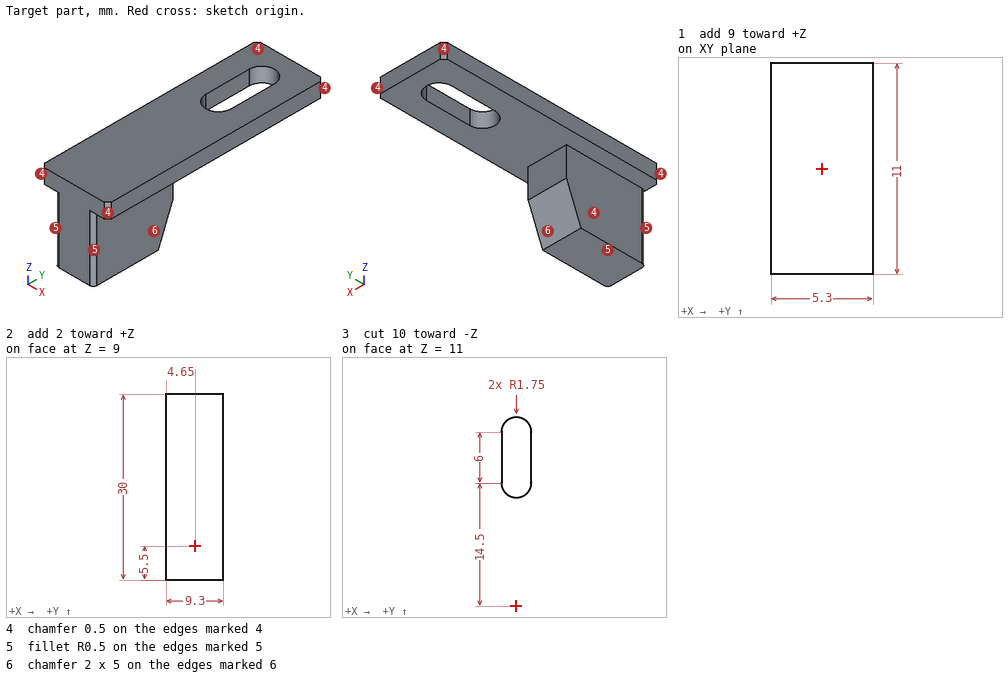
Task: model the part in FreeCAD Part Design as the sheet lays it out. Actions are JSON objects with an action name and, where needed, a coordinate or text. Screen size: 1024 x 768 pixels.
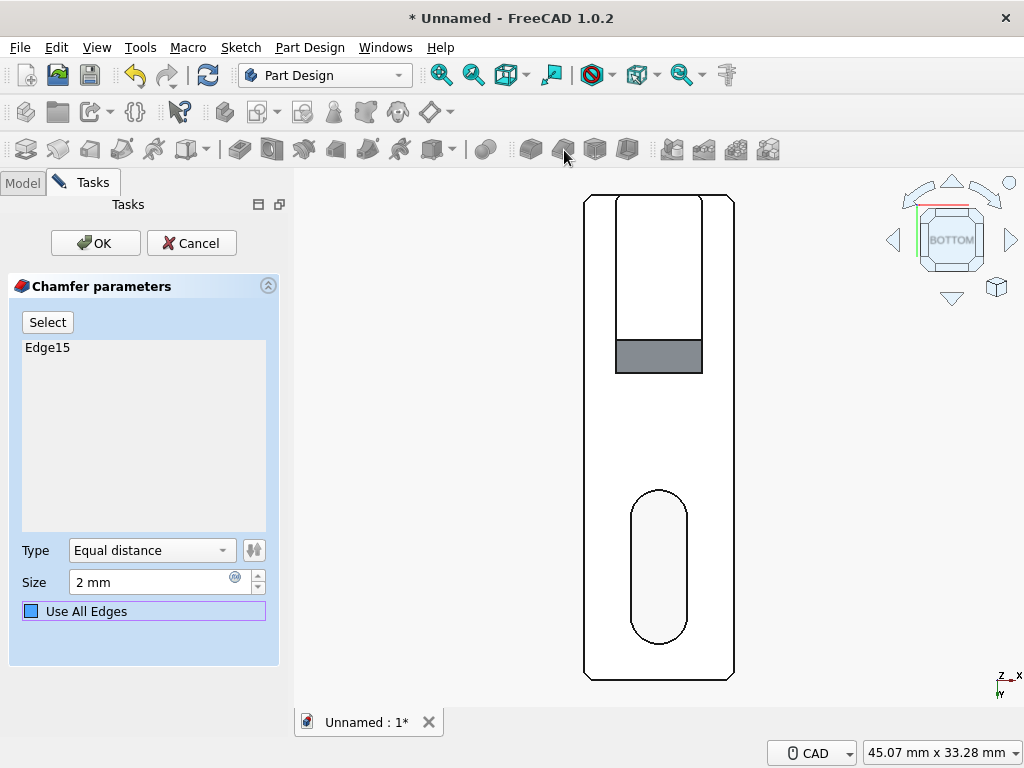
{"action": "left_click", "coordinate": [153, 550]}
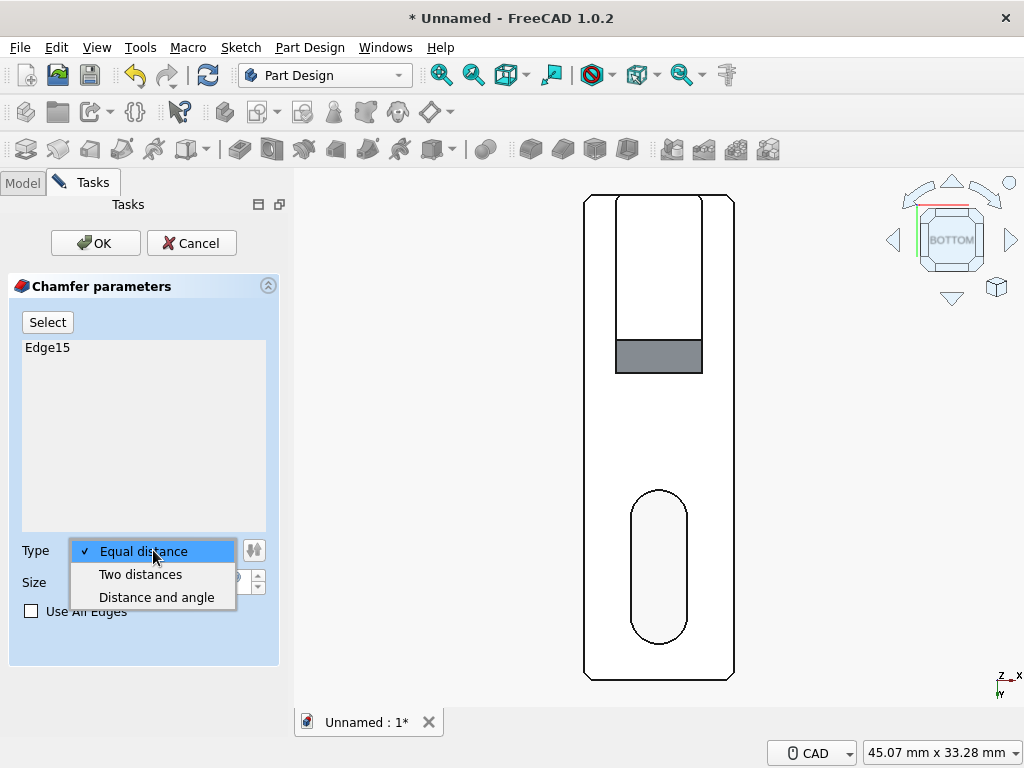
{"action": "left_click", "coordinate": [152, 574]}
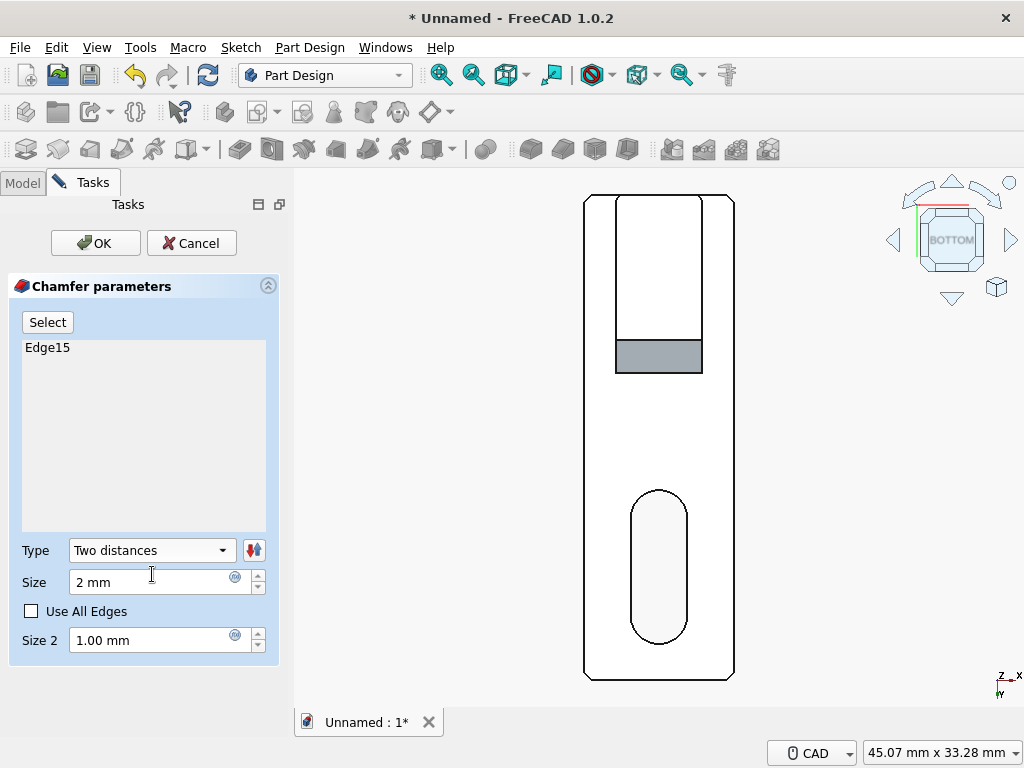
{"action": "triple_click", "coordinate": [160, 640]}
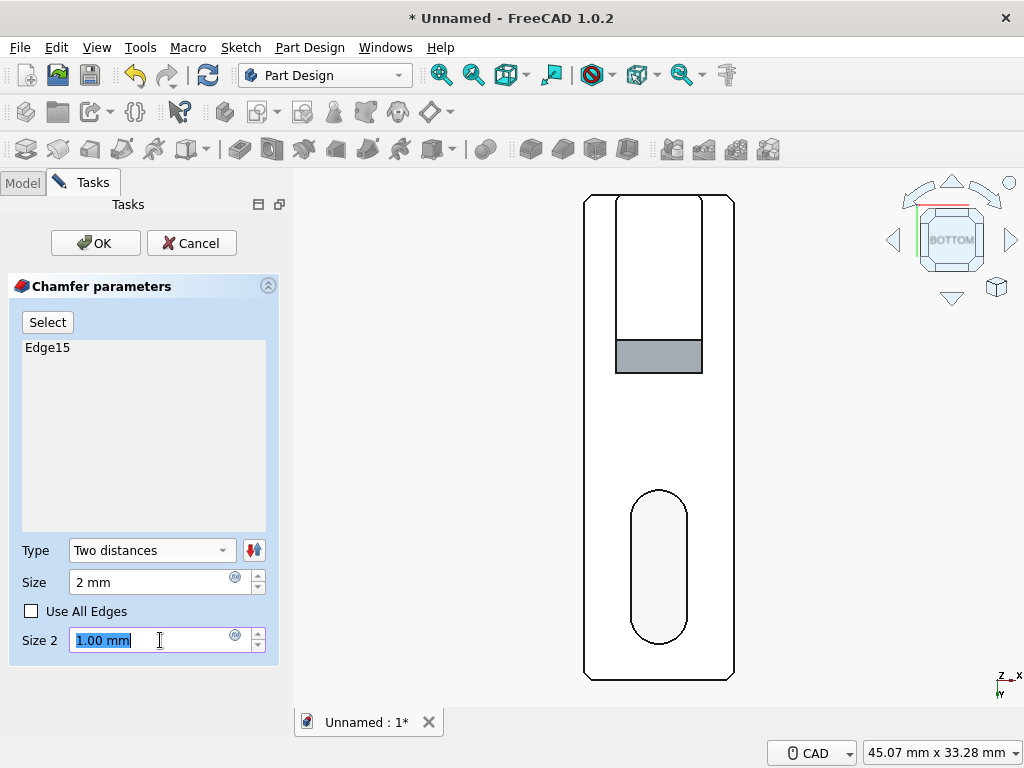
{"action": "type", "text": "5"}
{"action": "key", "text": "Tab"}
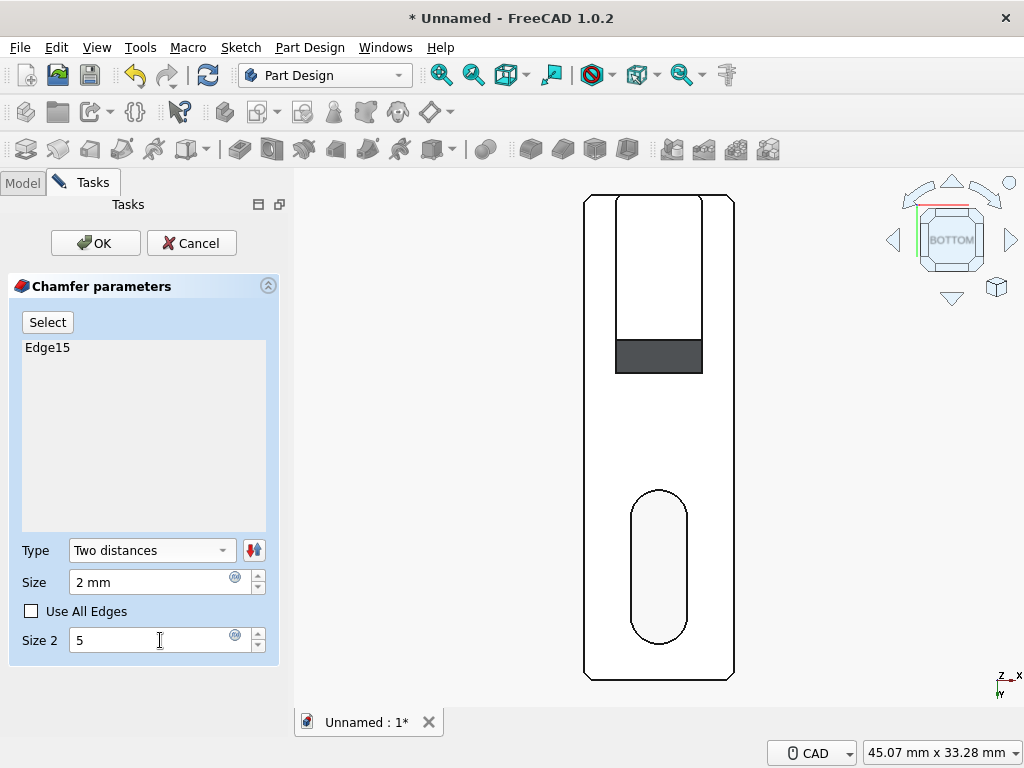
{"action": "left_click", "coordinate": [96, 243]}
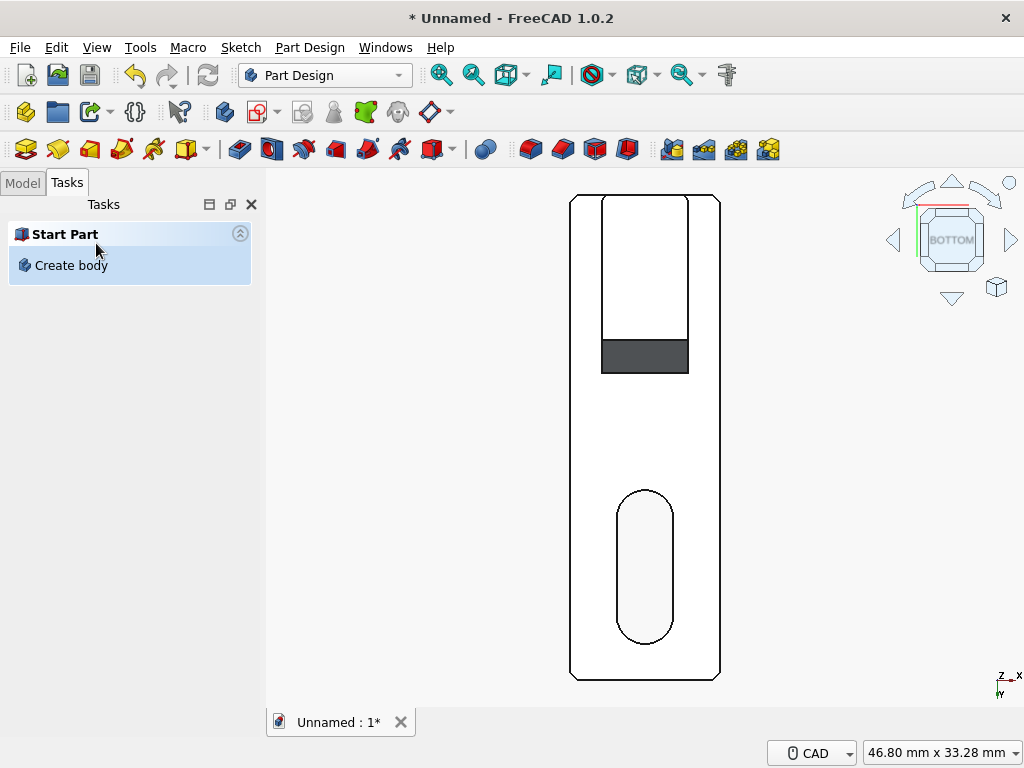
{"action": "key", "text": "0"}